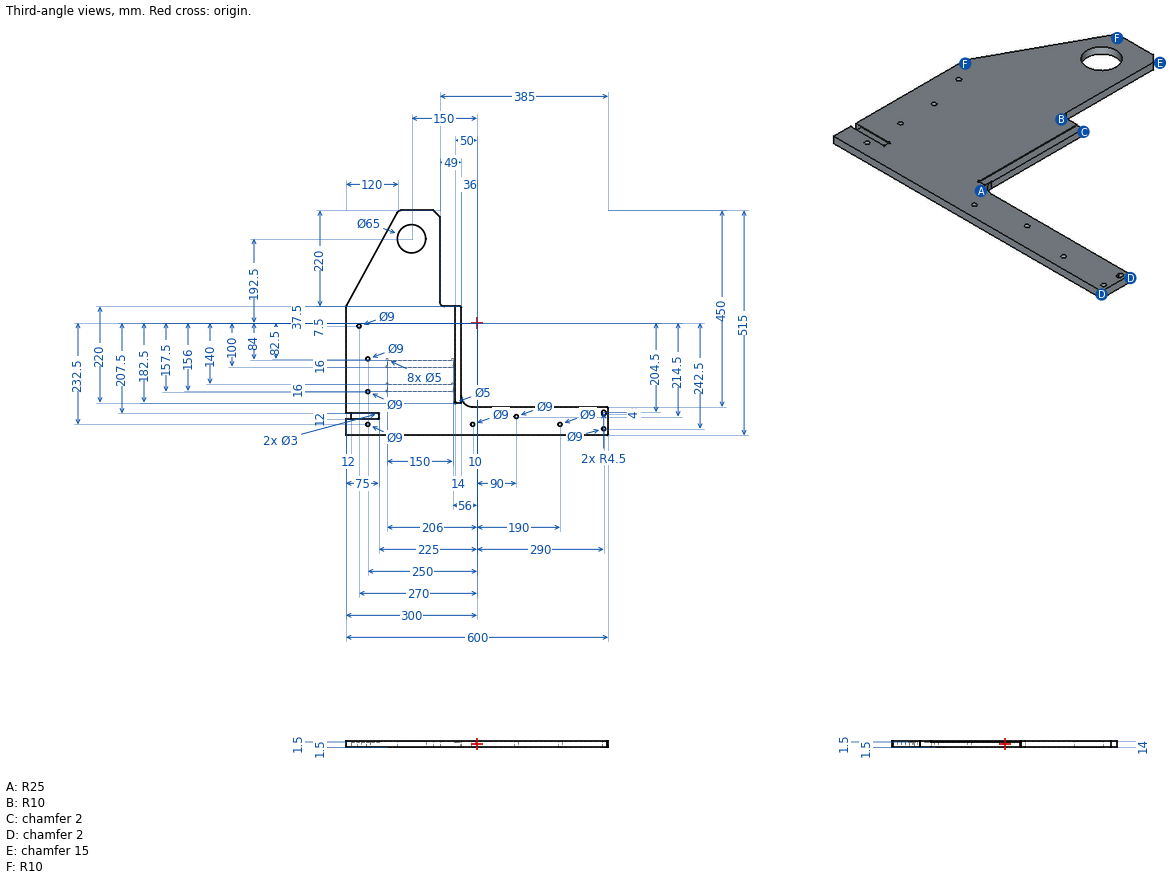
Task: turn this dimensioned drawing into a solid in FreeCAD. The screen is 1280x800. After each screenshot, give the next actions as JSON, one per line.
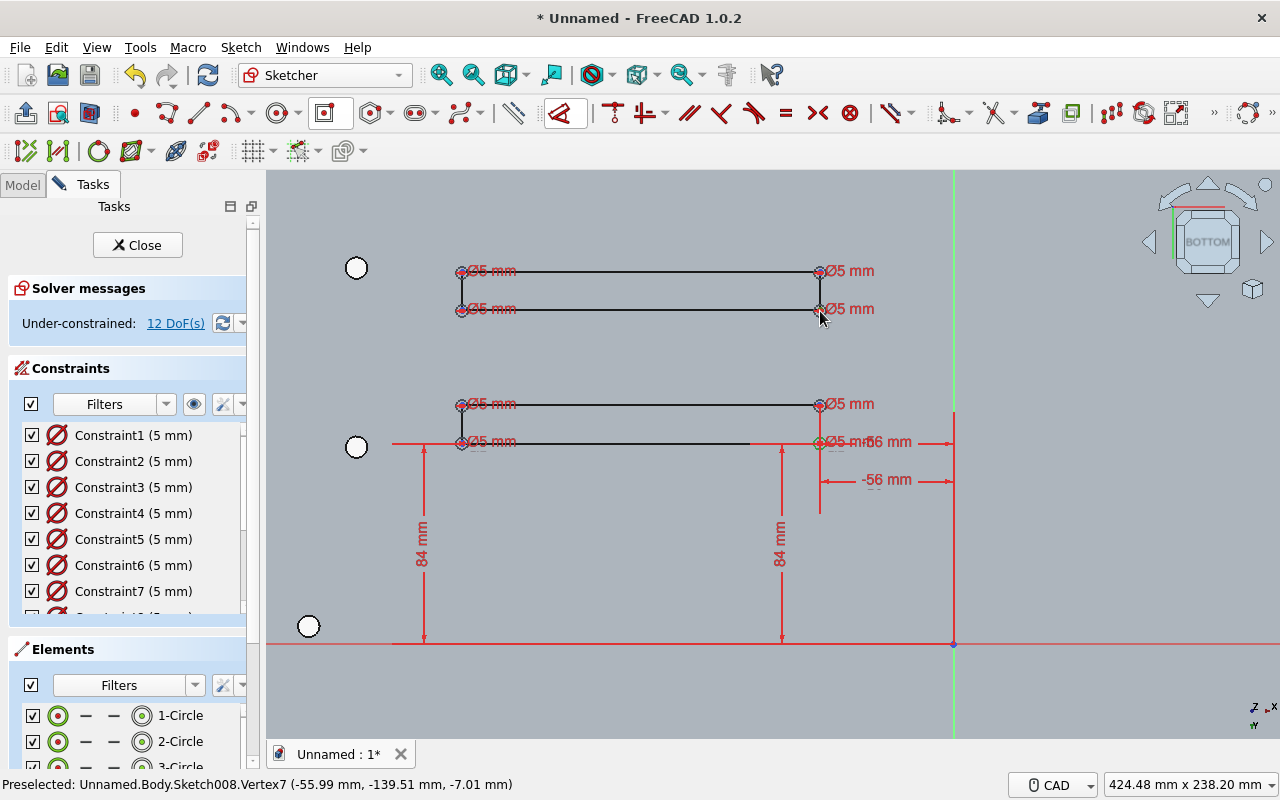
{"action": "key", "text": "l"}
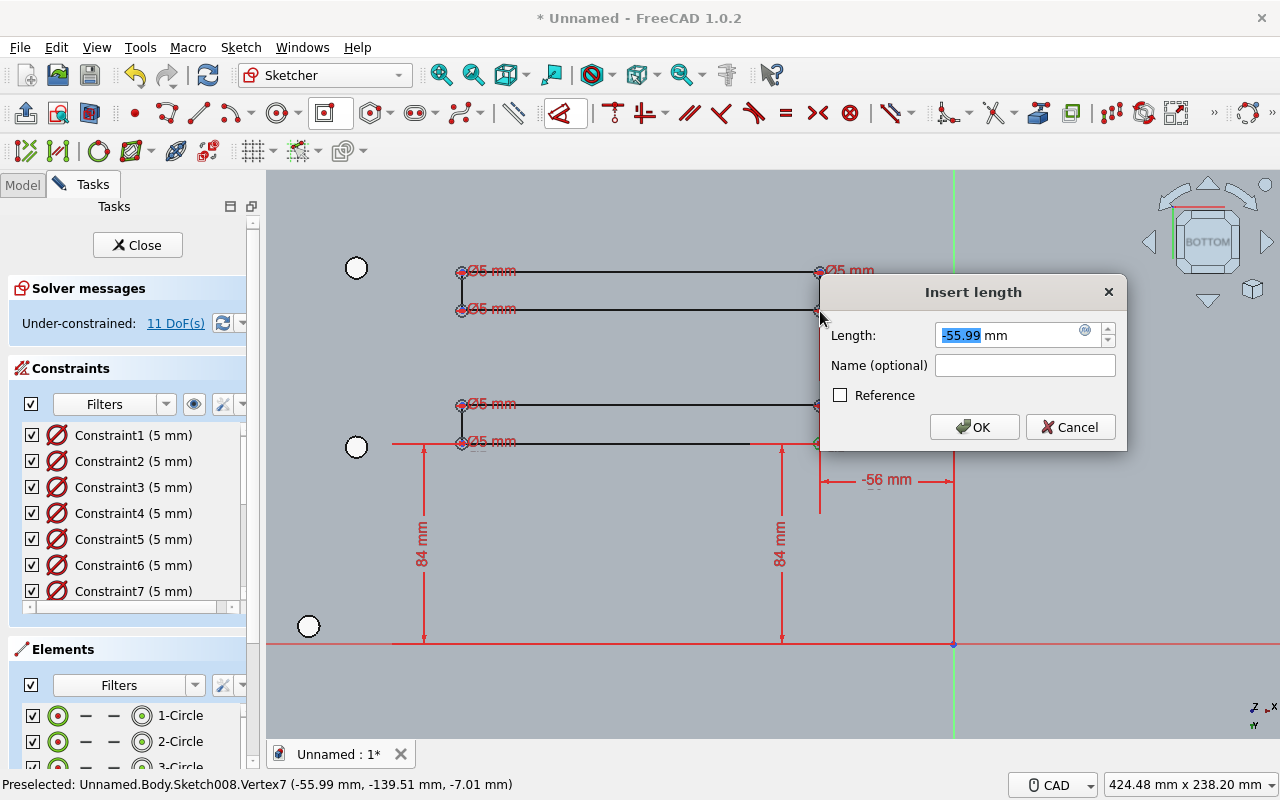
{"action": "type", "text": "-56"}
{"action": "key", "text": "Return"}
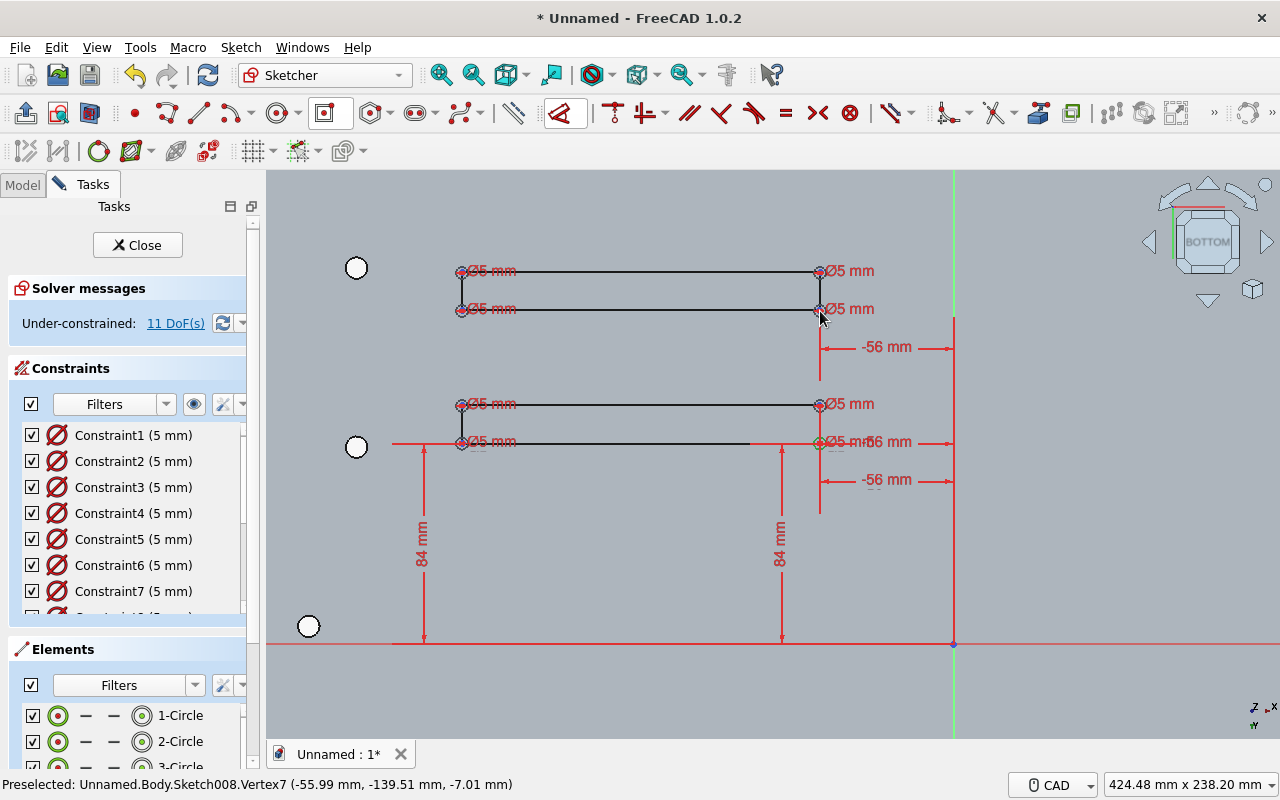
{"action": "left_click", "coordinate": [820, 273]}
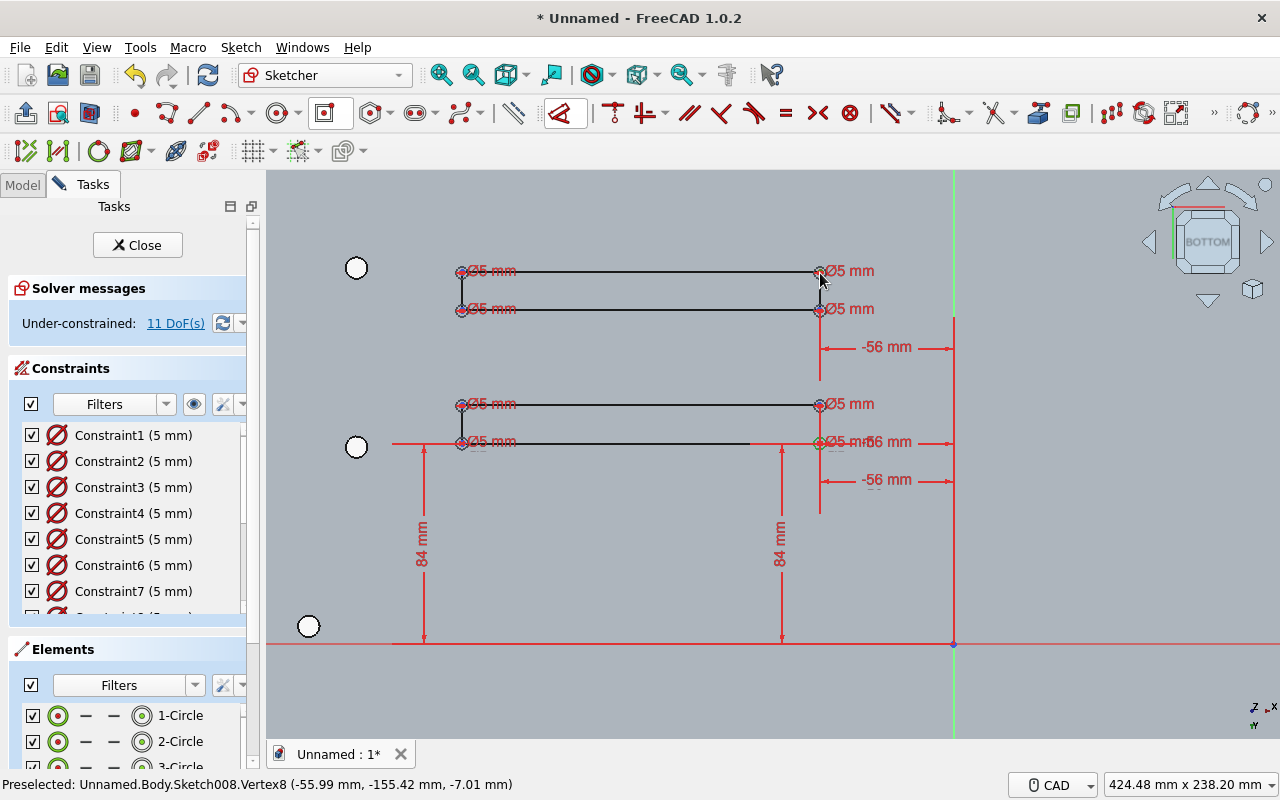
{"action": "key", "text": "l"}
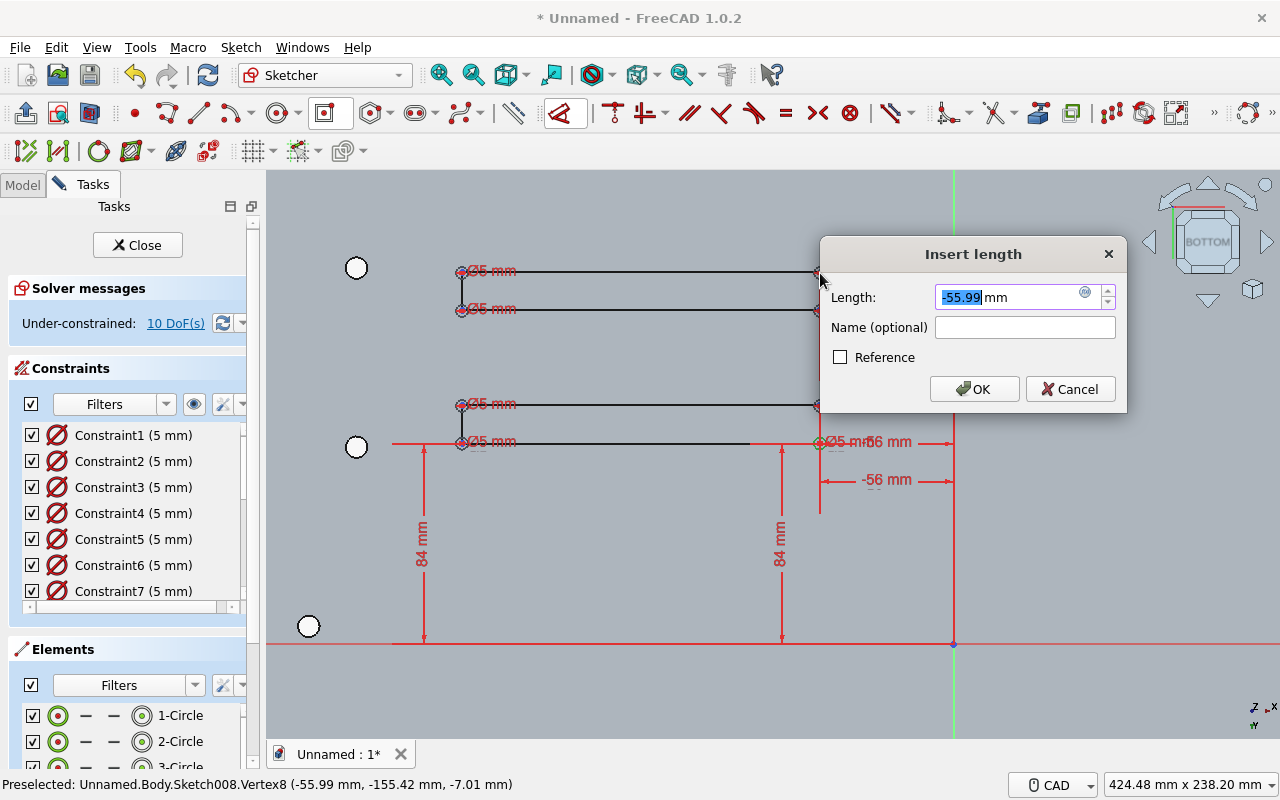
{"action": "type", "text": "-56"}
{"action": "key", "text": "Return"}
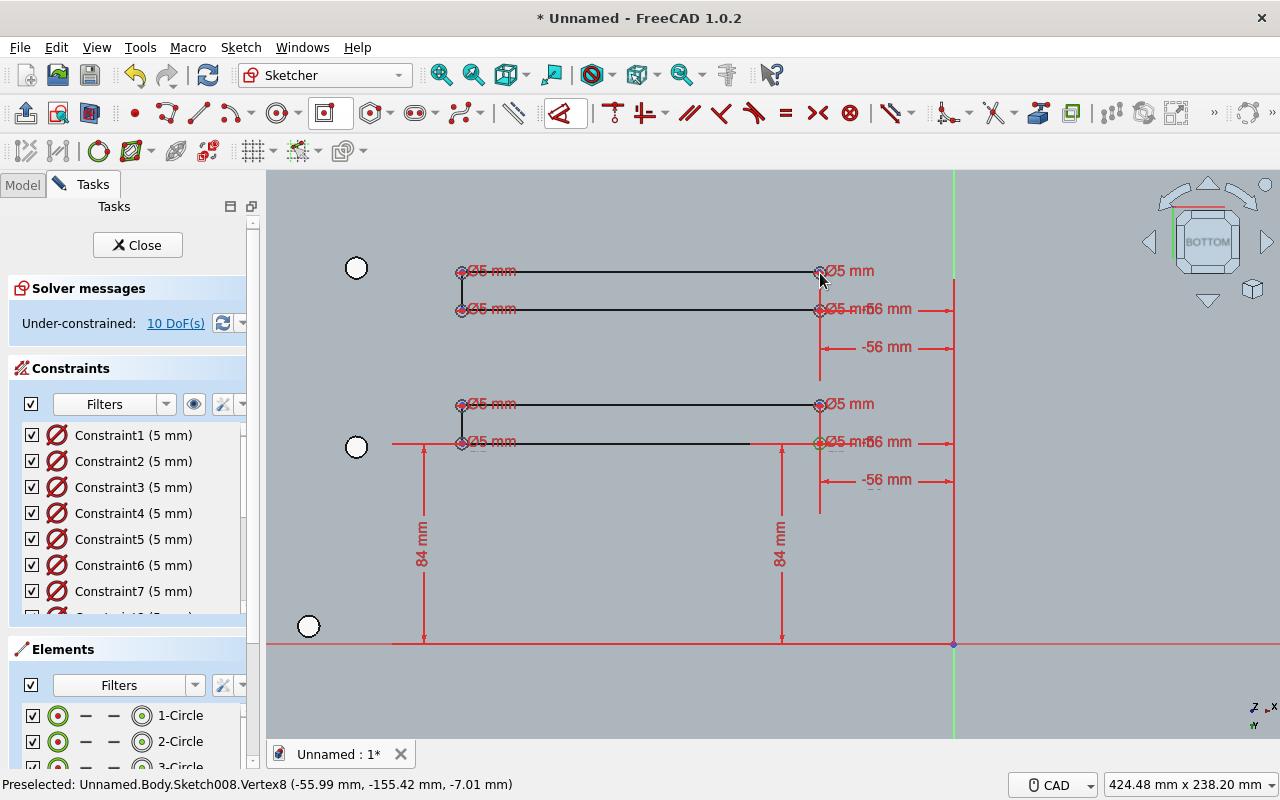
{"action": "left_click", "coordinate": [462, 444]}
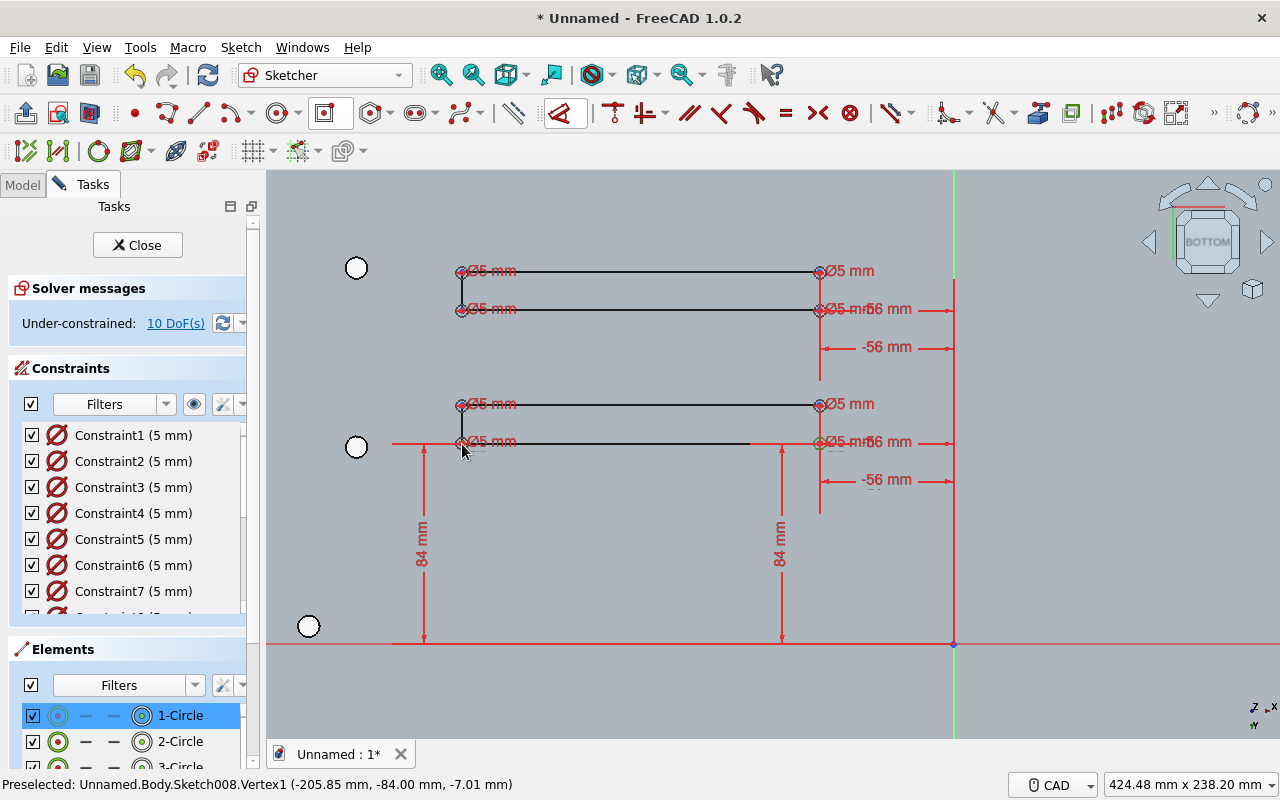
{"action": "left_click", "coordinate": [582, 114]}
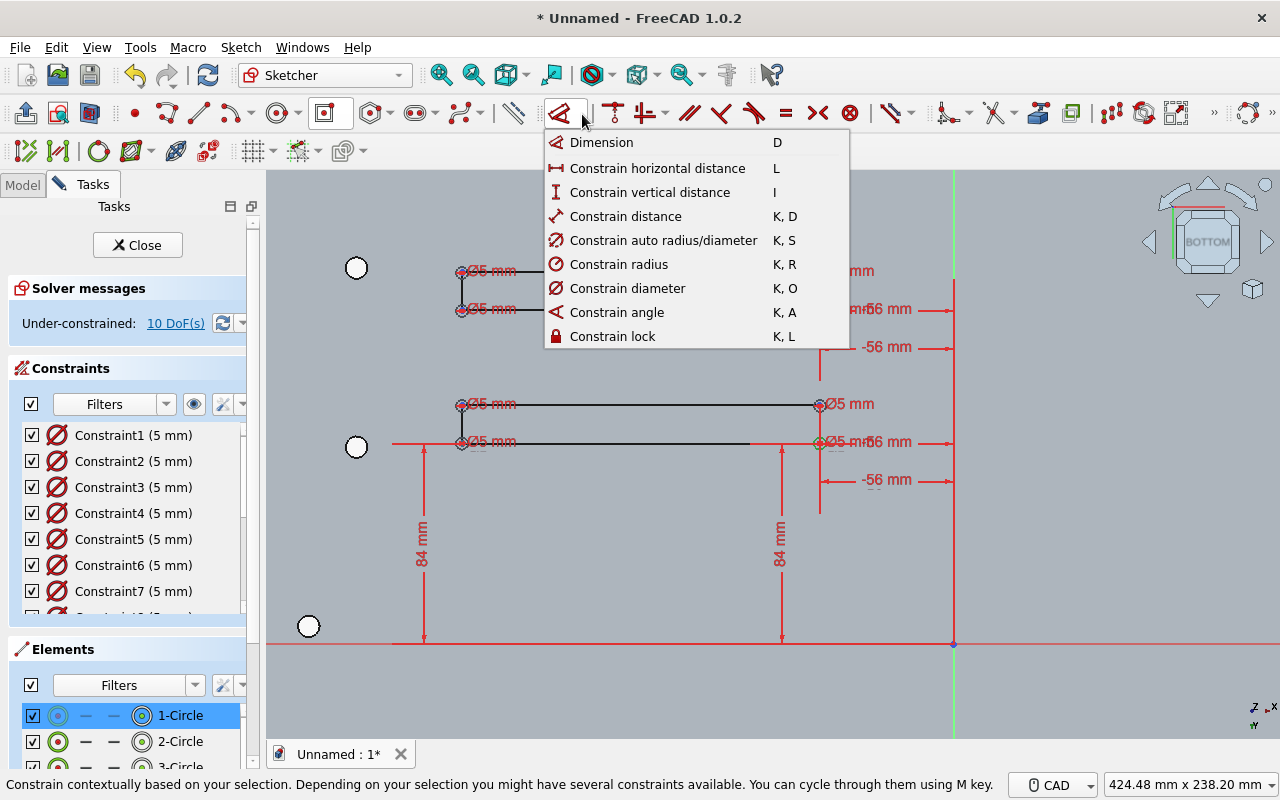
{"action": "left_click", "coordinate": [697, 168]}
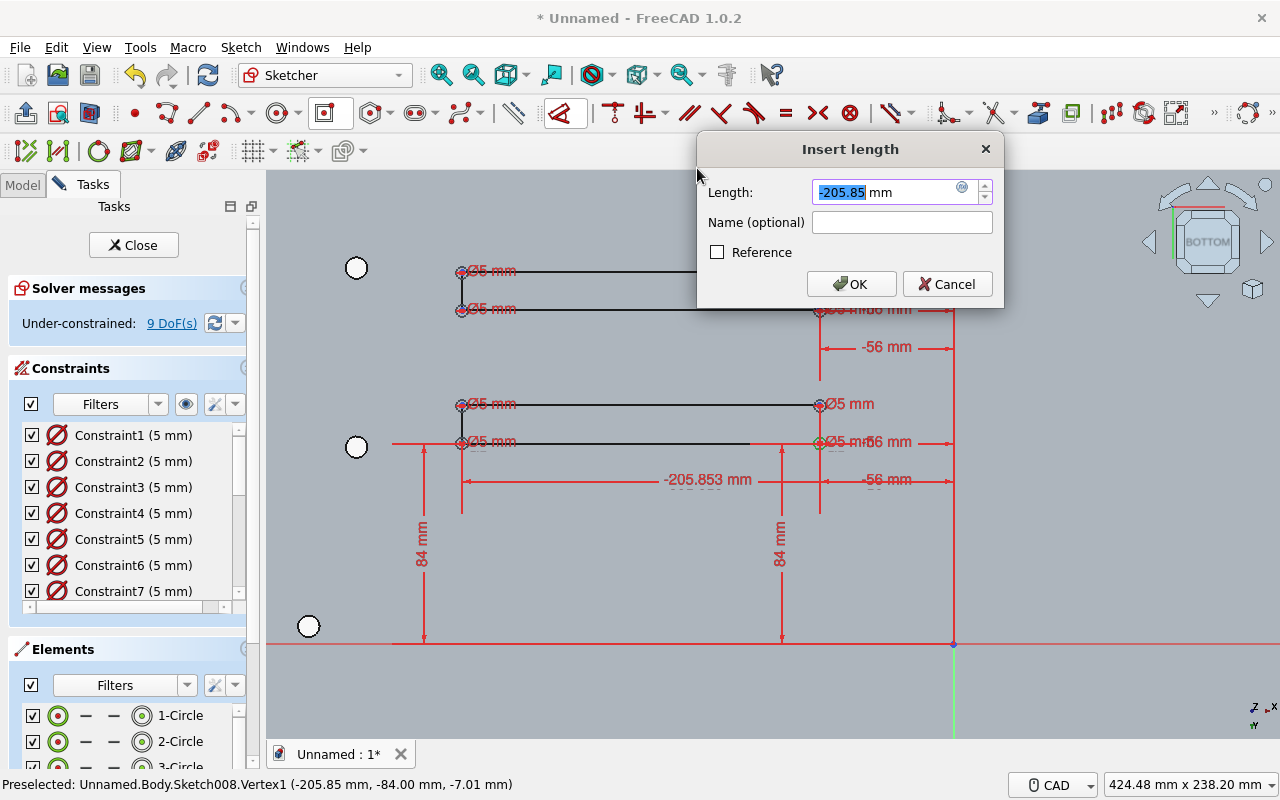
{"action": "type", "text": "-206"}
{"action": "key", "text": "Return"}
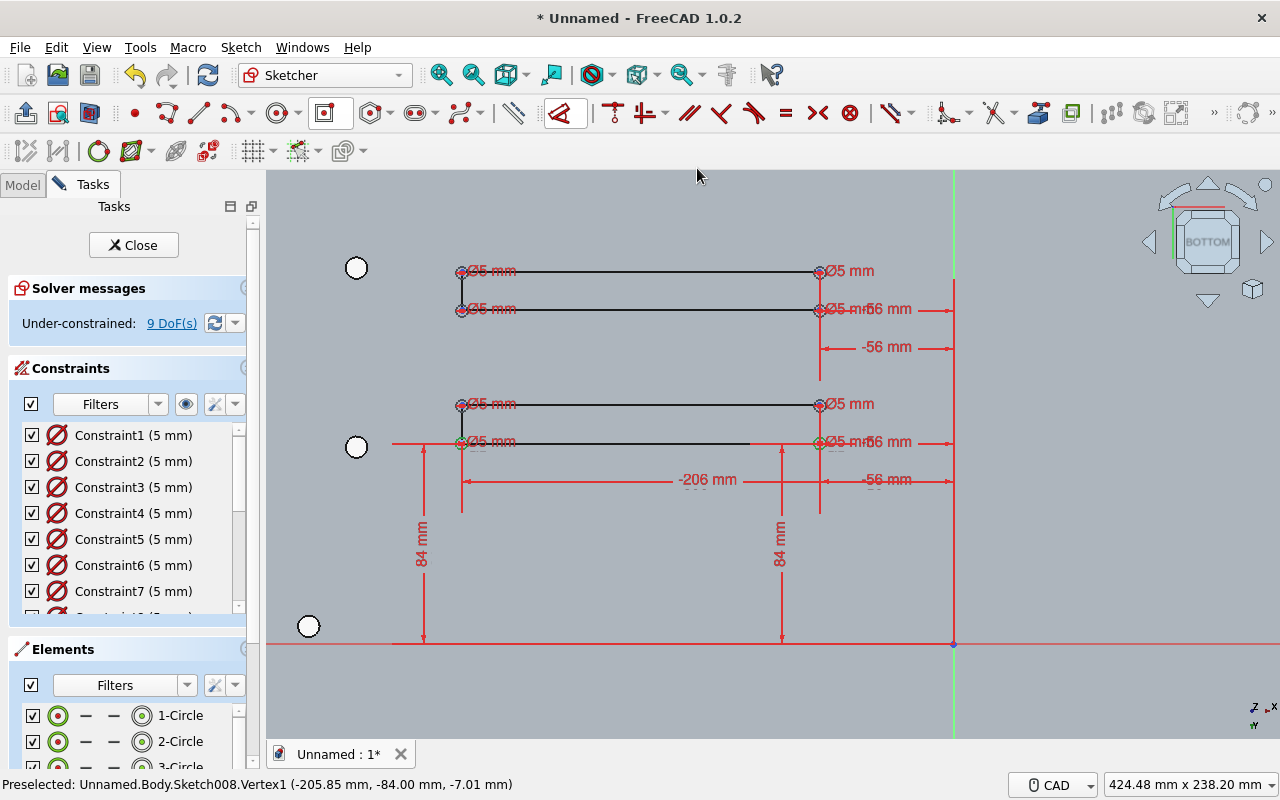
{"action": "left_click", "coordinate": [462, 406]}